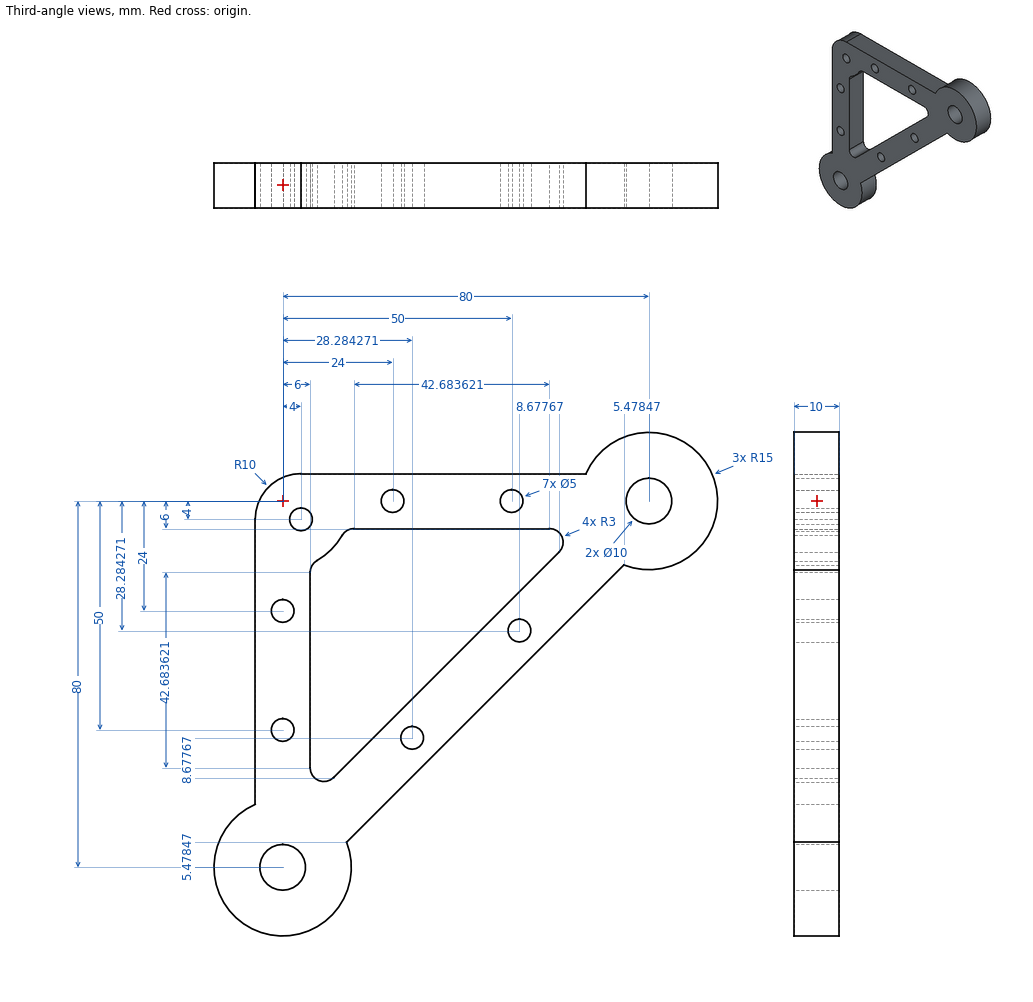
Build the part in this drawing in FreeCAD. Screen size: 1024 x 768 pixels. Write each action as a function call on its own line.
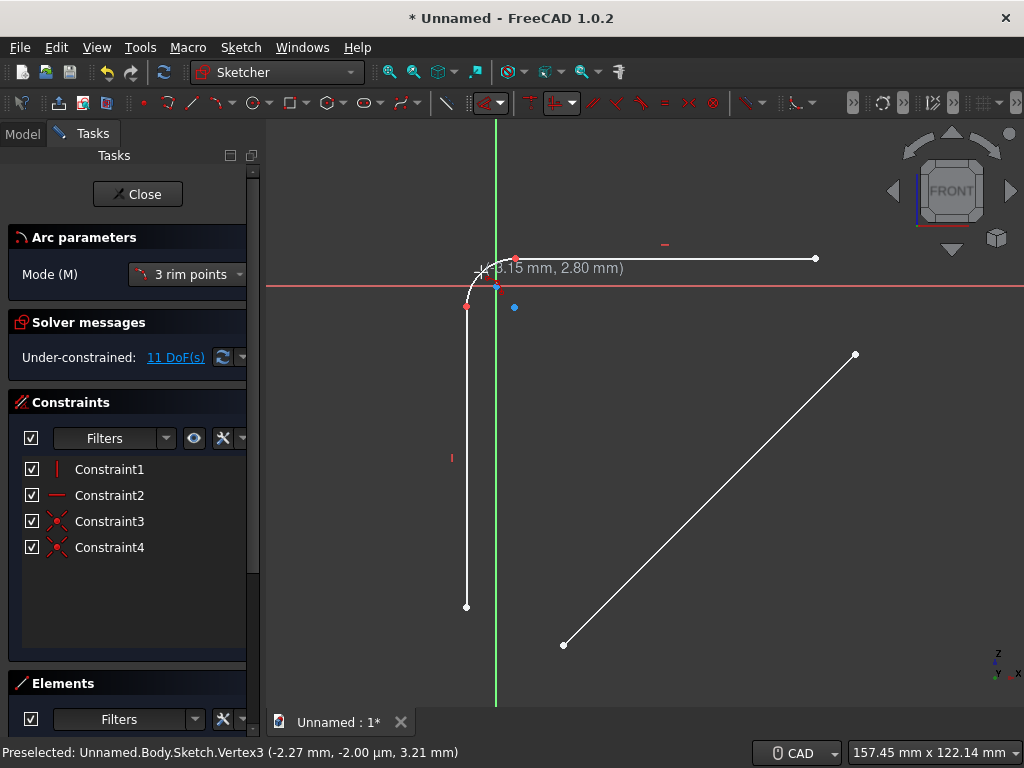
click(815, 259)
click(855, 355)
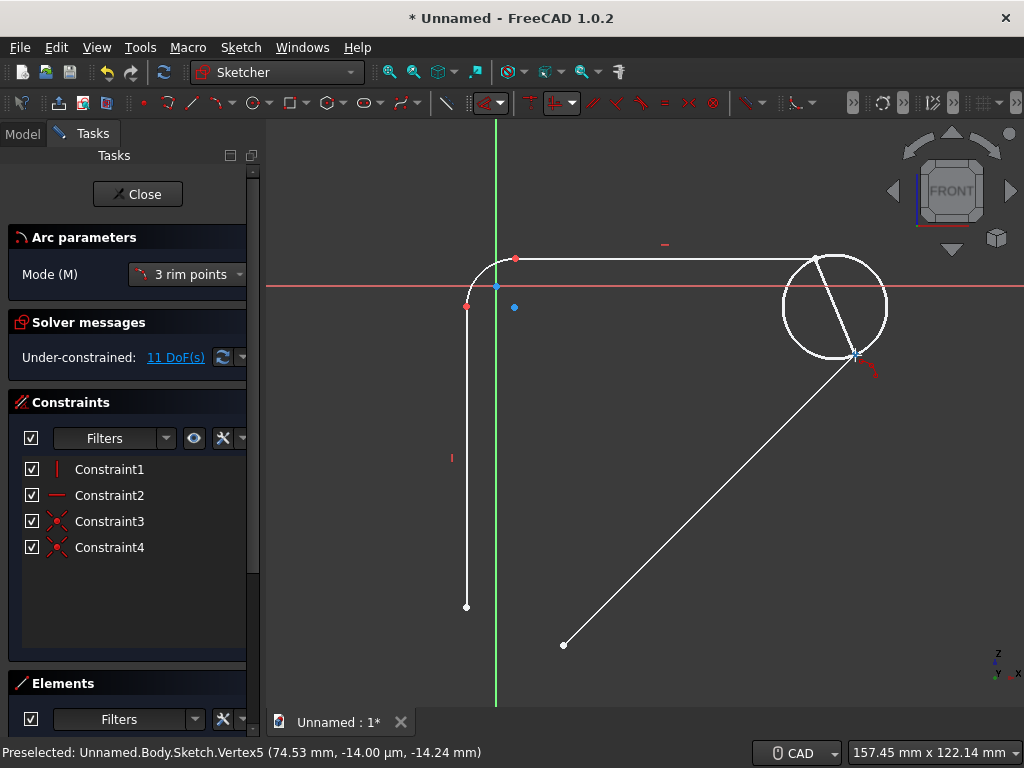
scroll(294, 147, down, 1)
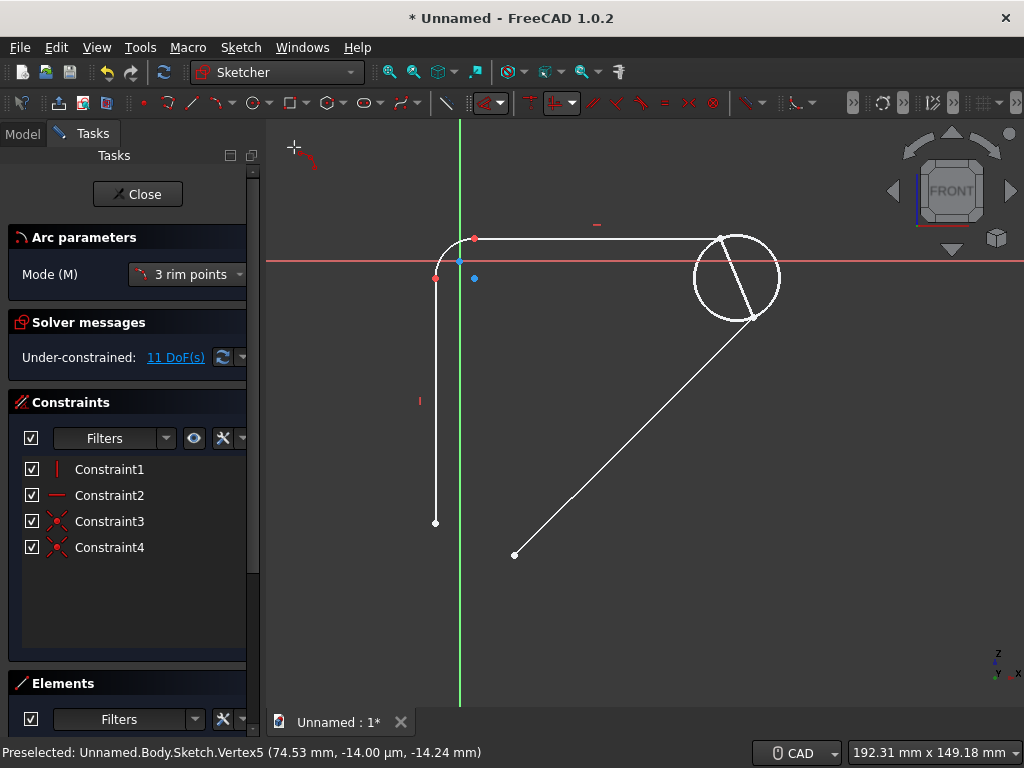
click(829, 239)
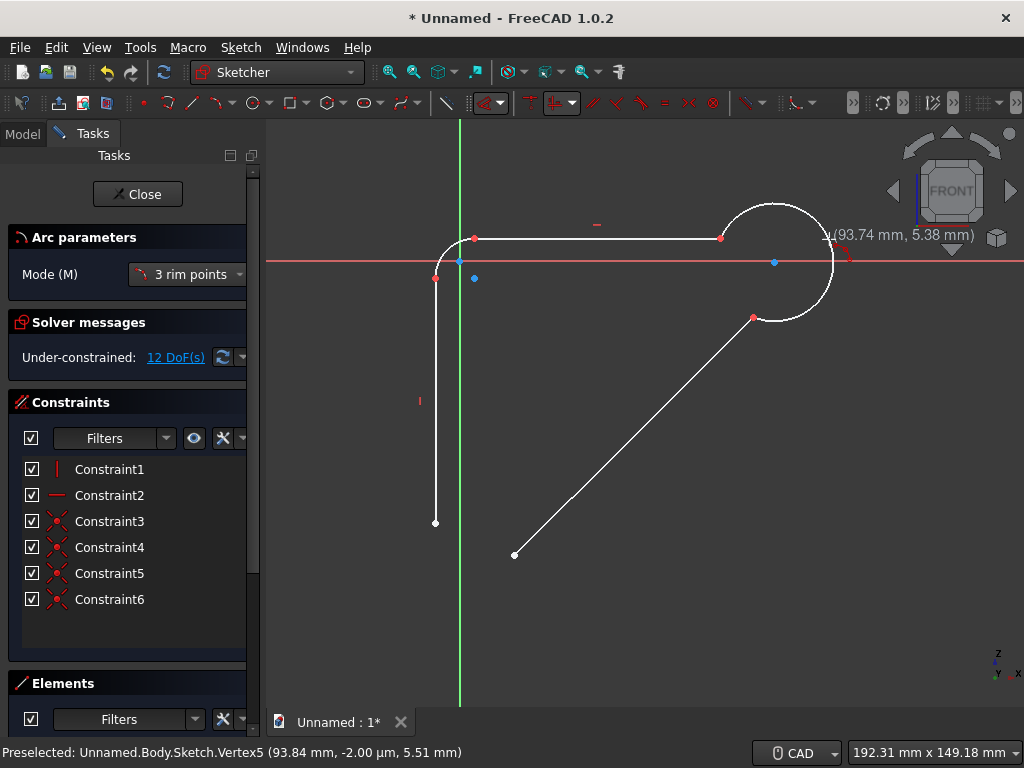
click(514, 556)
click(436, 524)
click(437, 631)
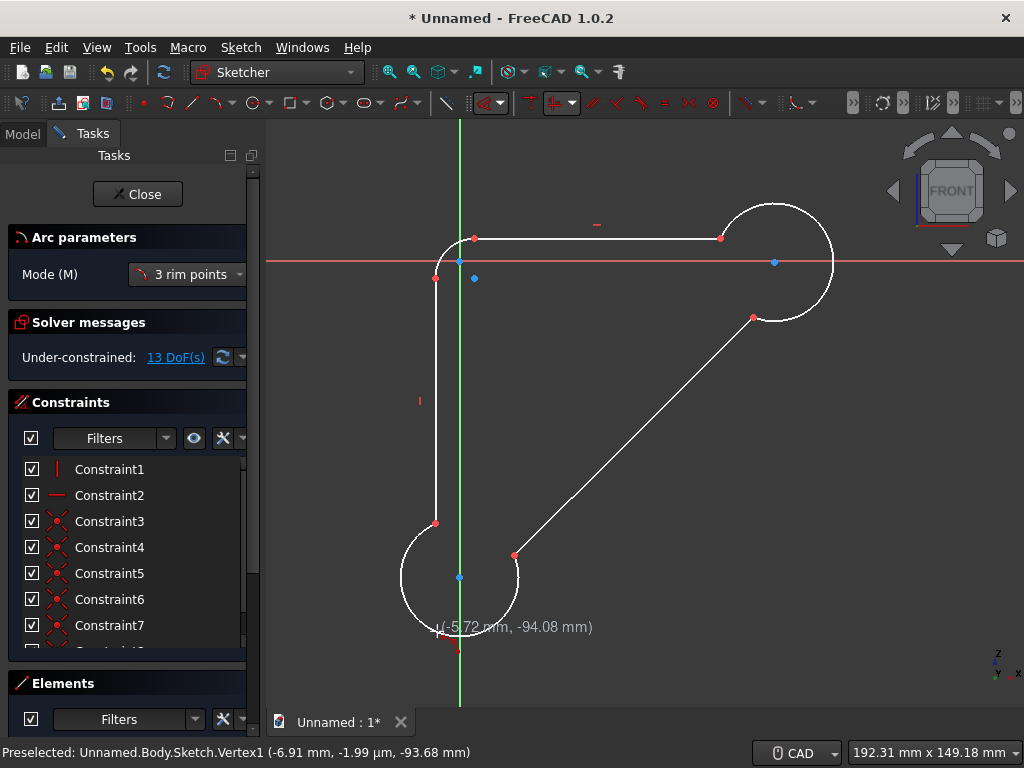
key(g)
key(l)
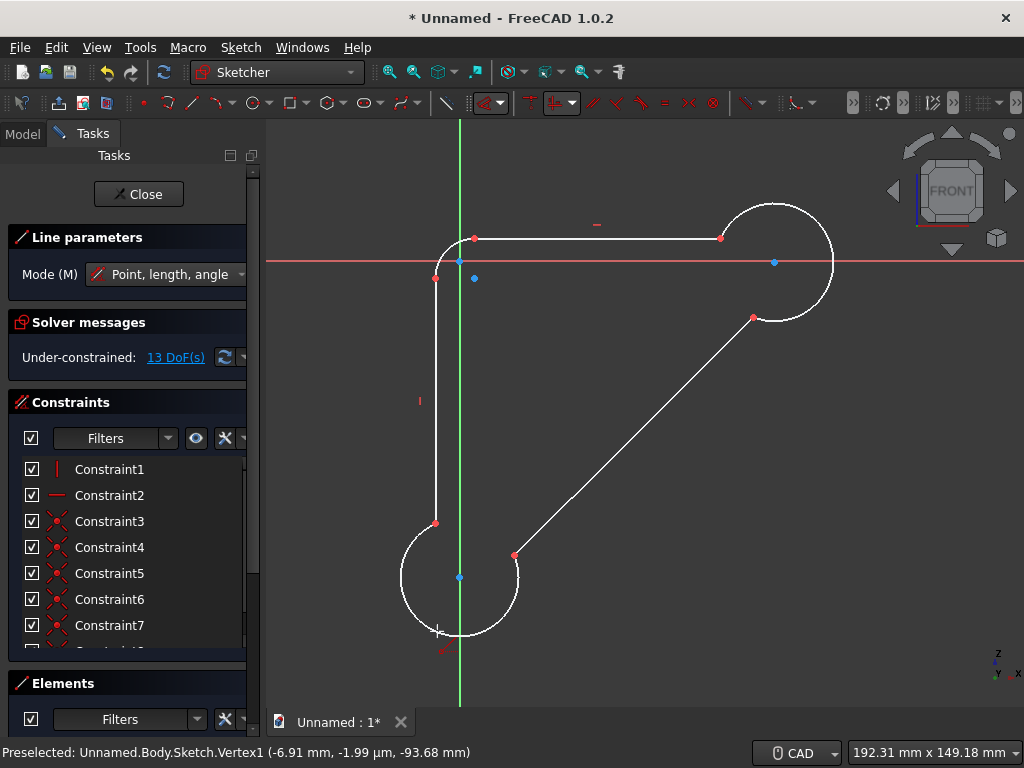
click(503, 499)
click(698, 305)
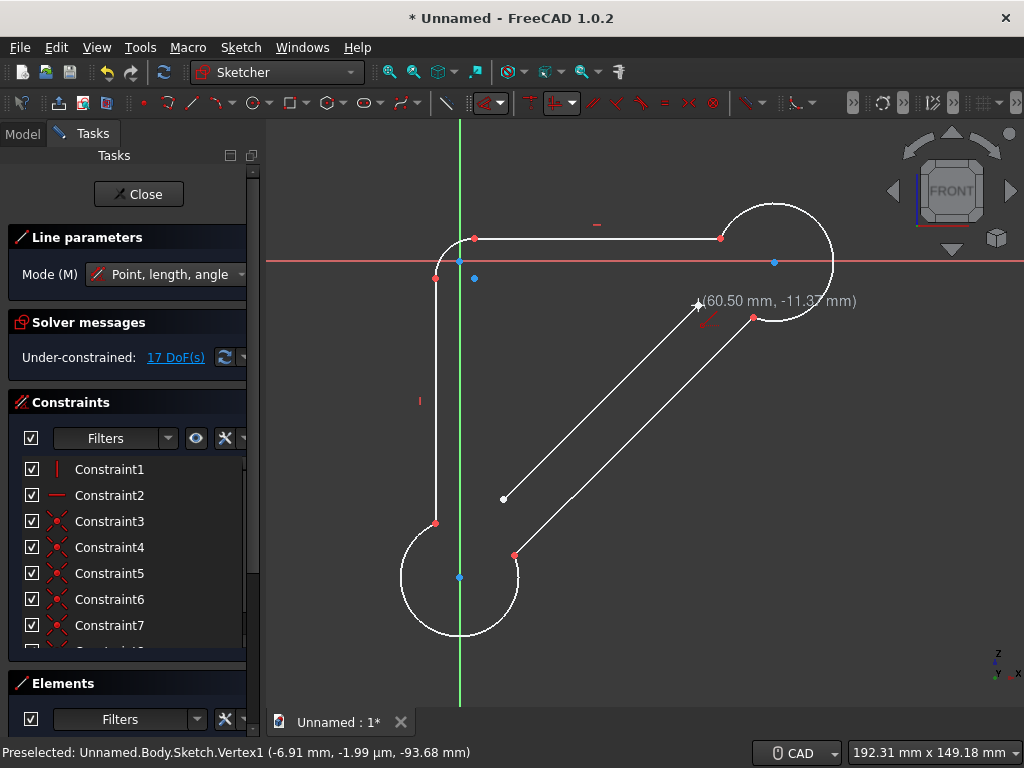
click(689, 285)
click(521, 285)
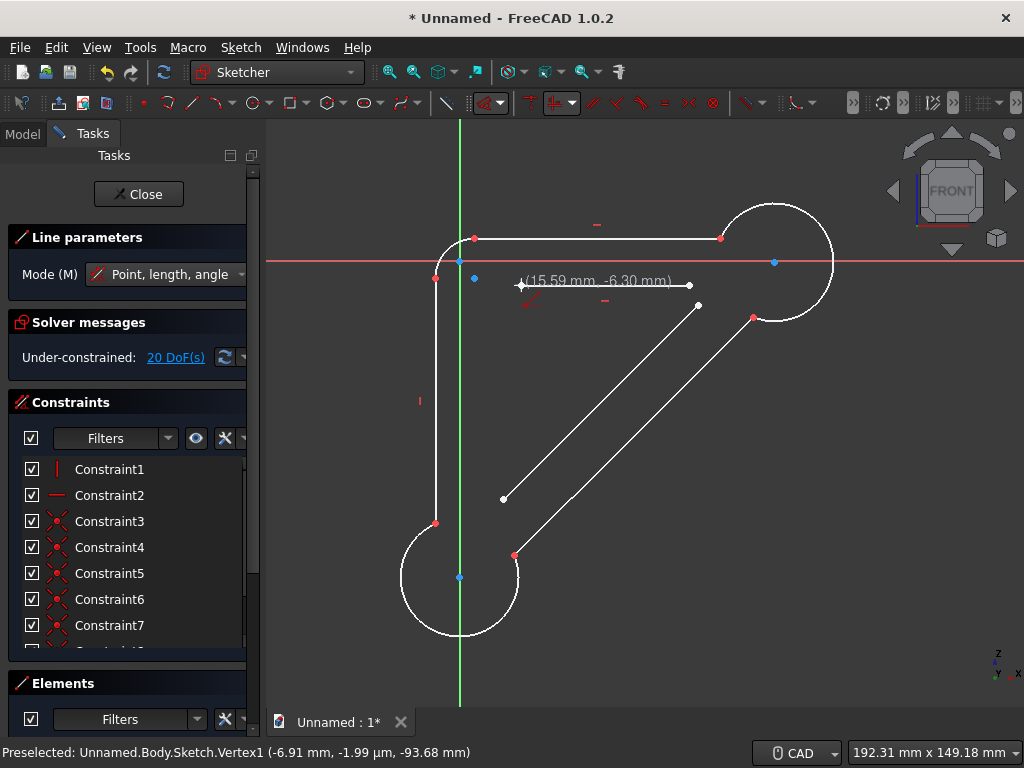
click(483, 323)
click(483, 491)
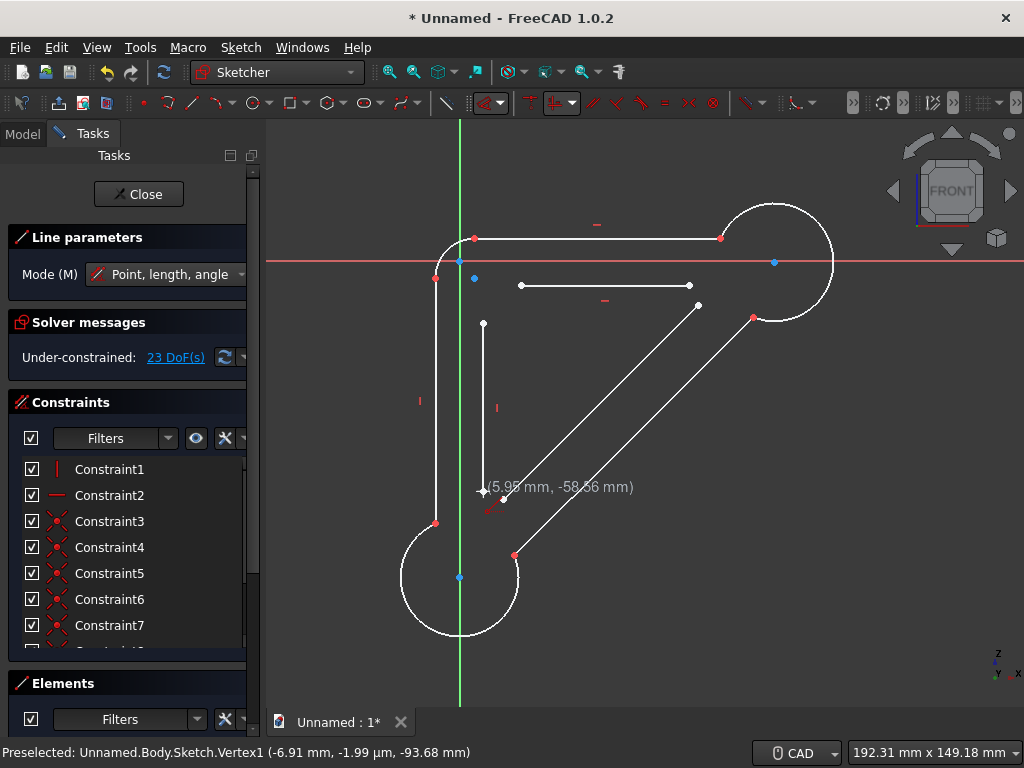
click(216, 104)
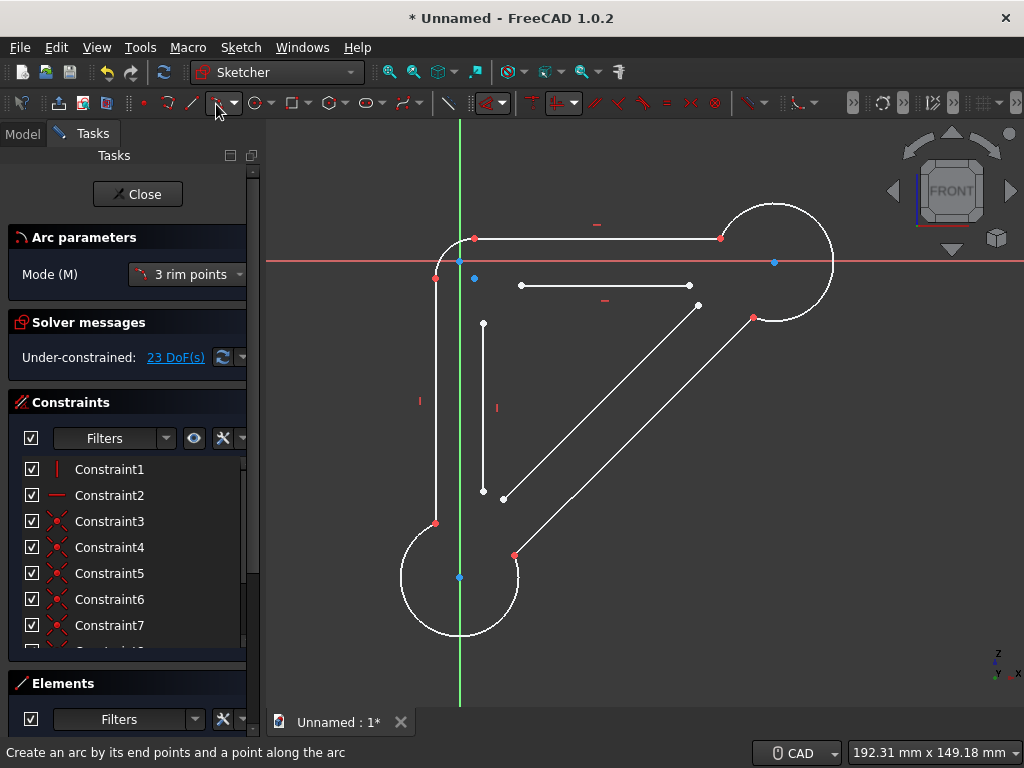
click(698, 306)
click(689, 286)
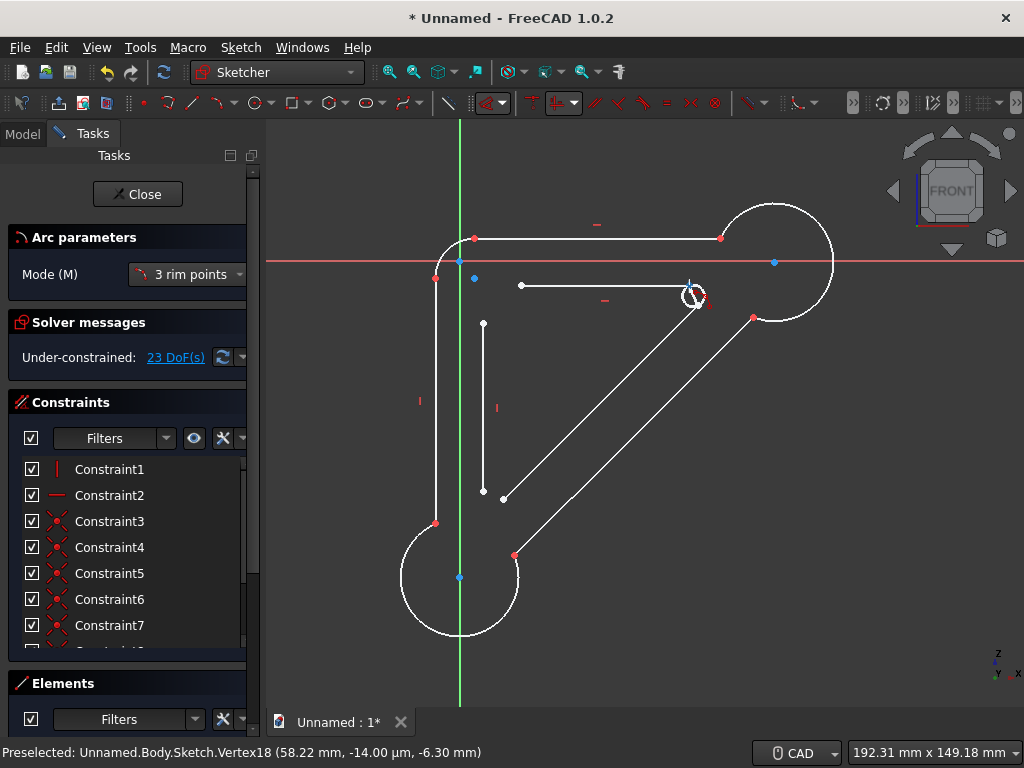
scroll(700, 292, up, 4)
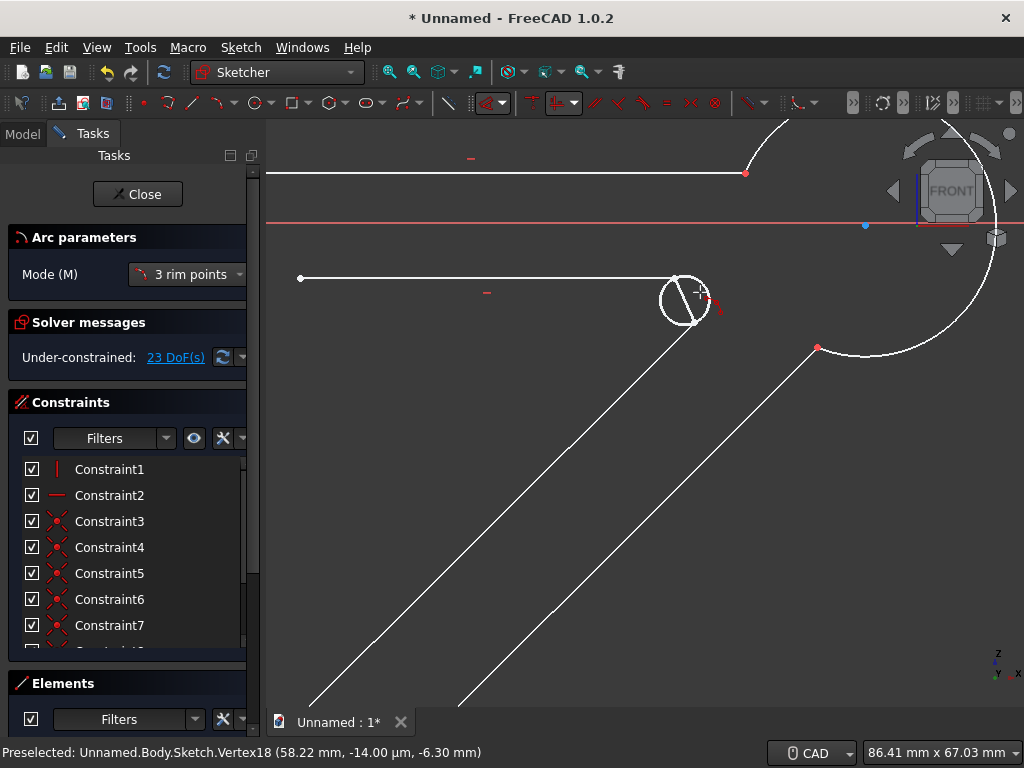
click(700, 292)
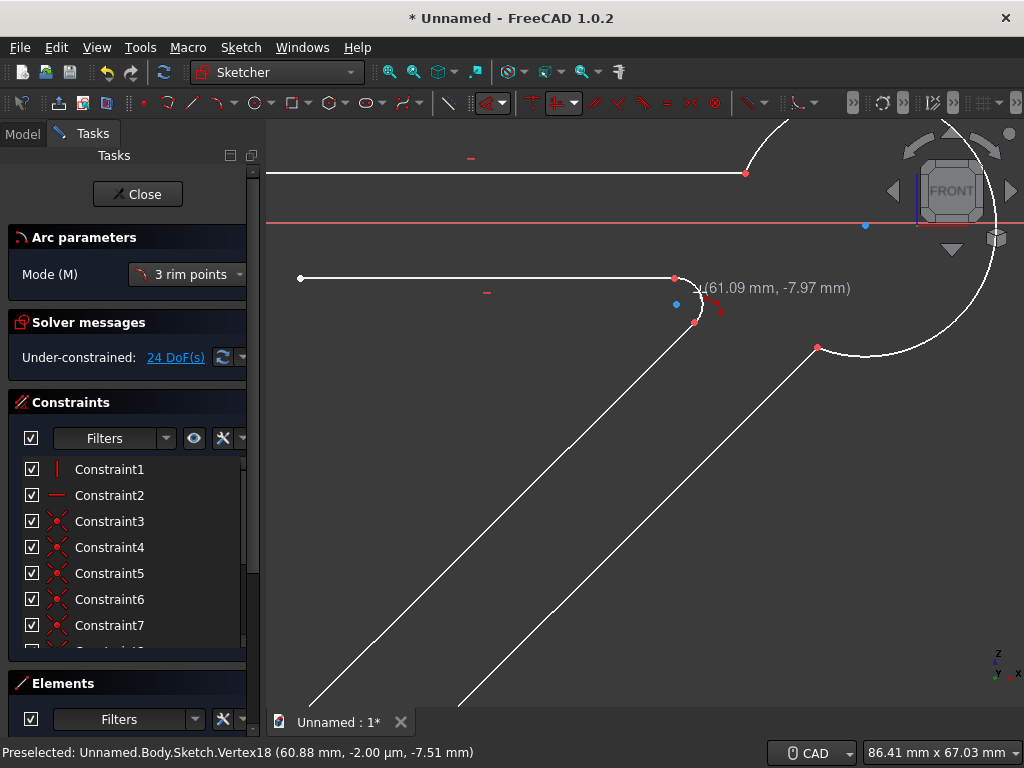
click(301, 278)